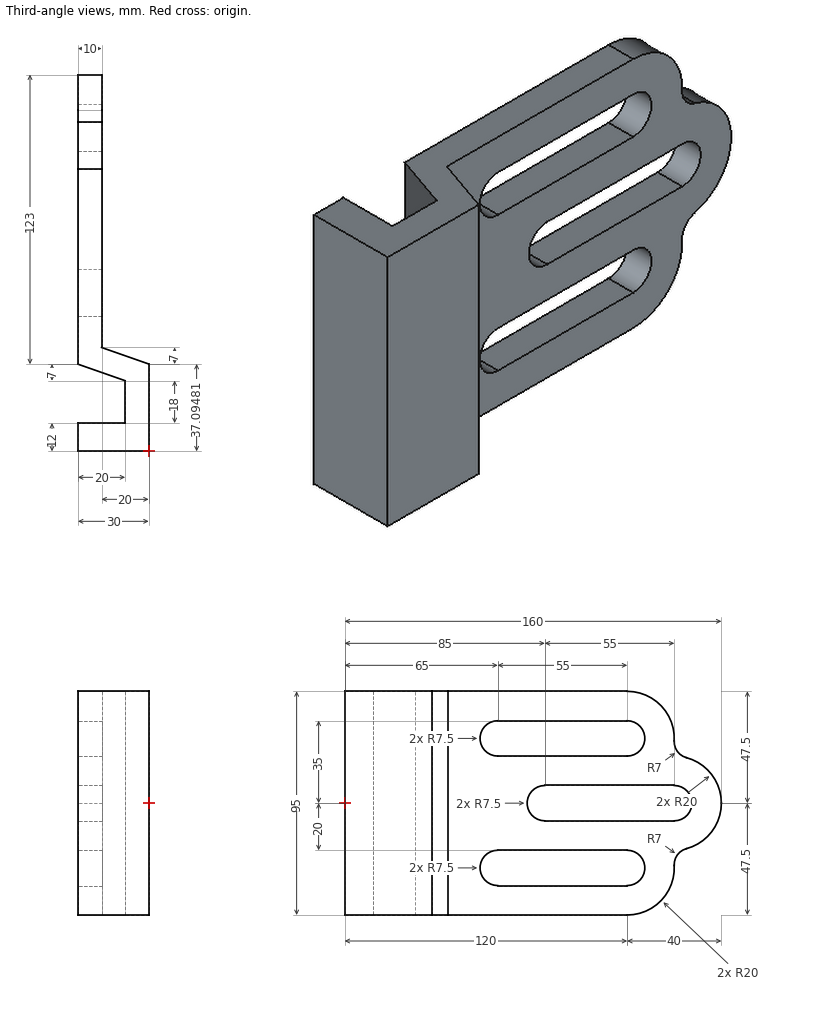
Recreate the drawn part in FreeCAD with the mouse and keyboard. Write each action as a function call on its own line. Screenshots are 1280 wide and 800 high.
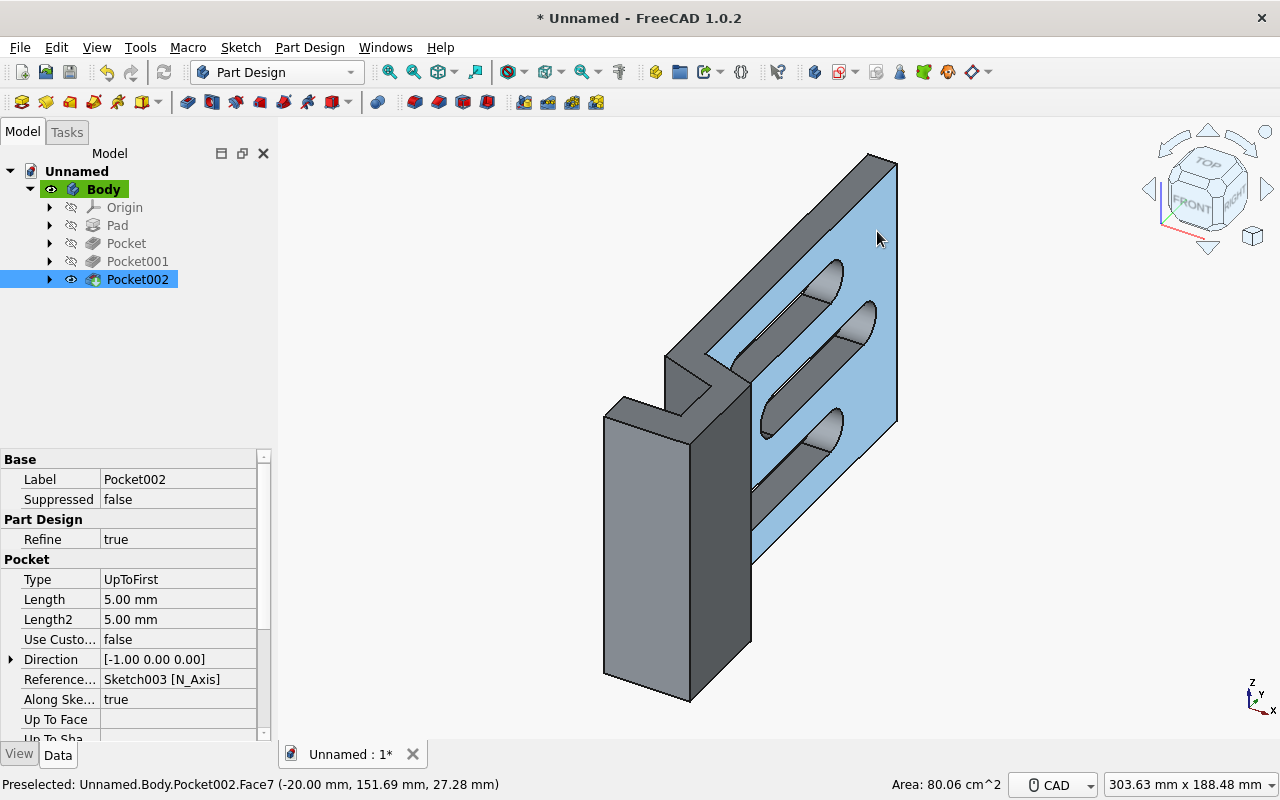
click(840, 72)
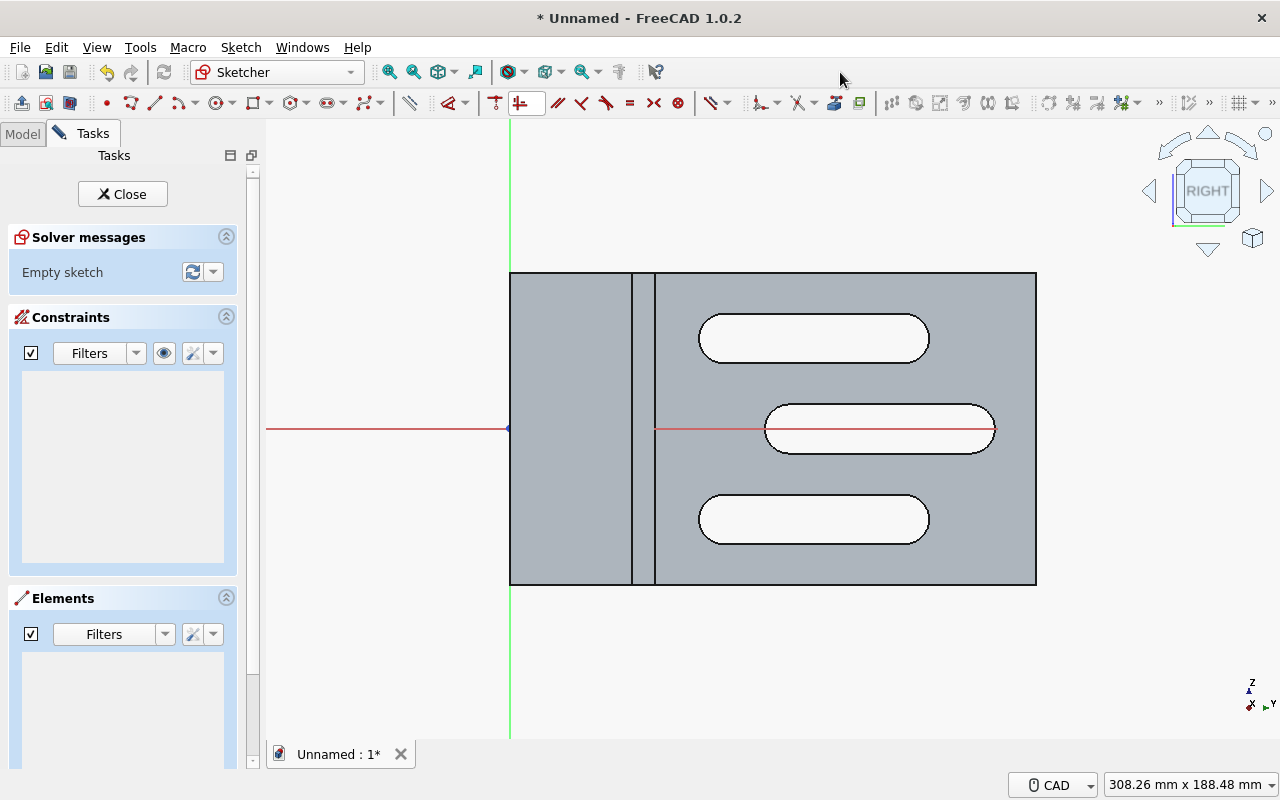
click(70, 104)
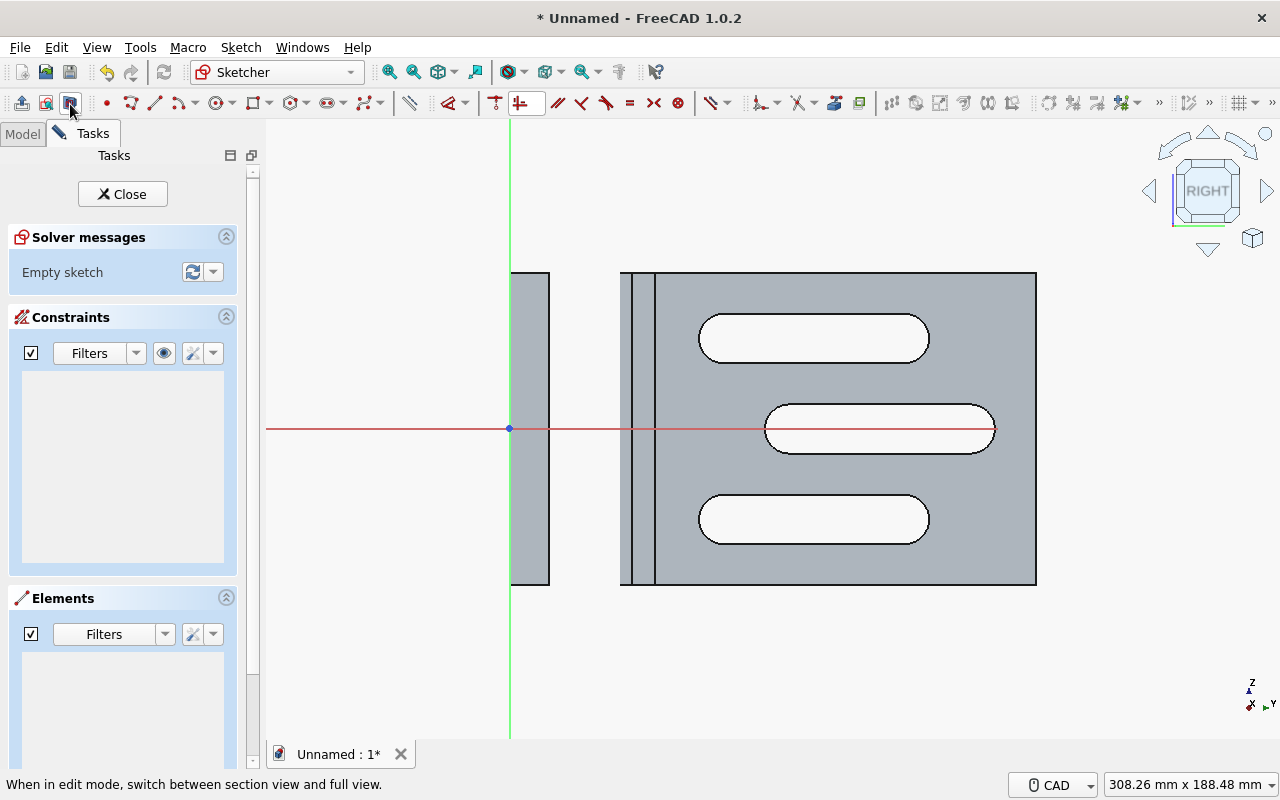
scroll(1115, 553, up, 5)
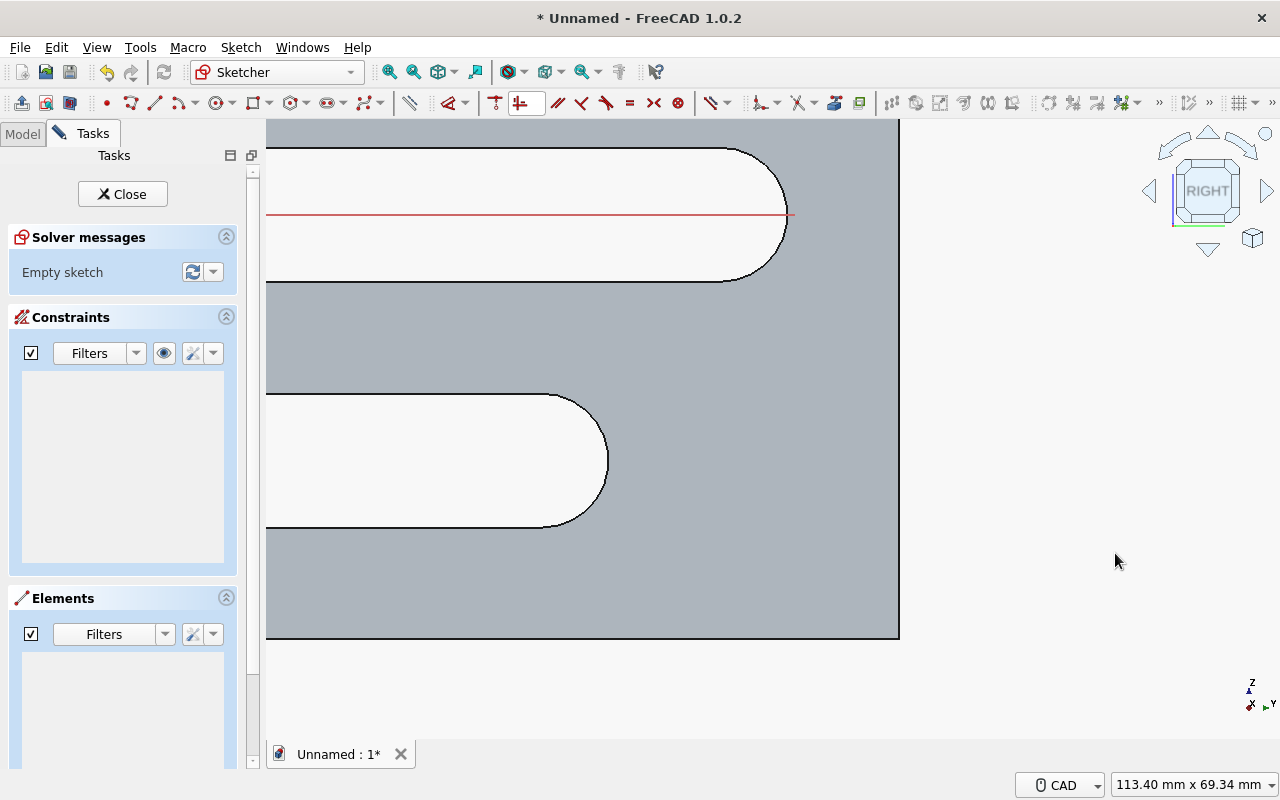
click(132, 104)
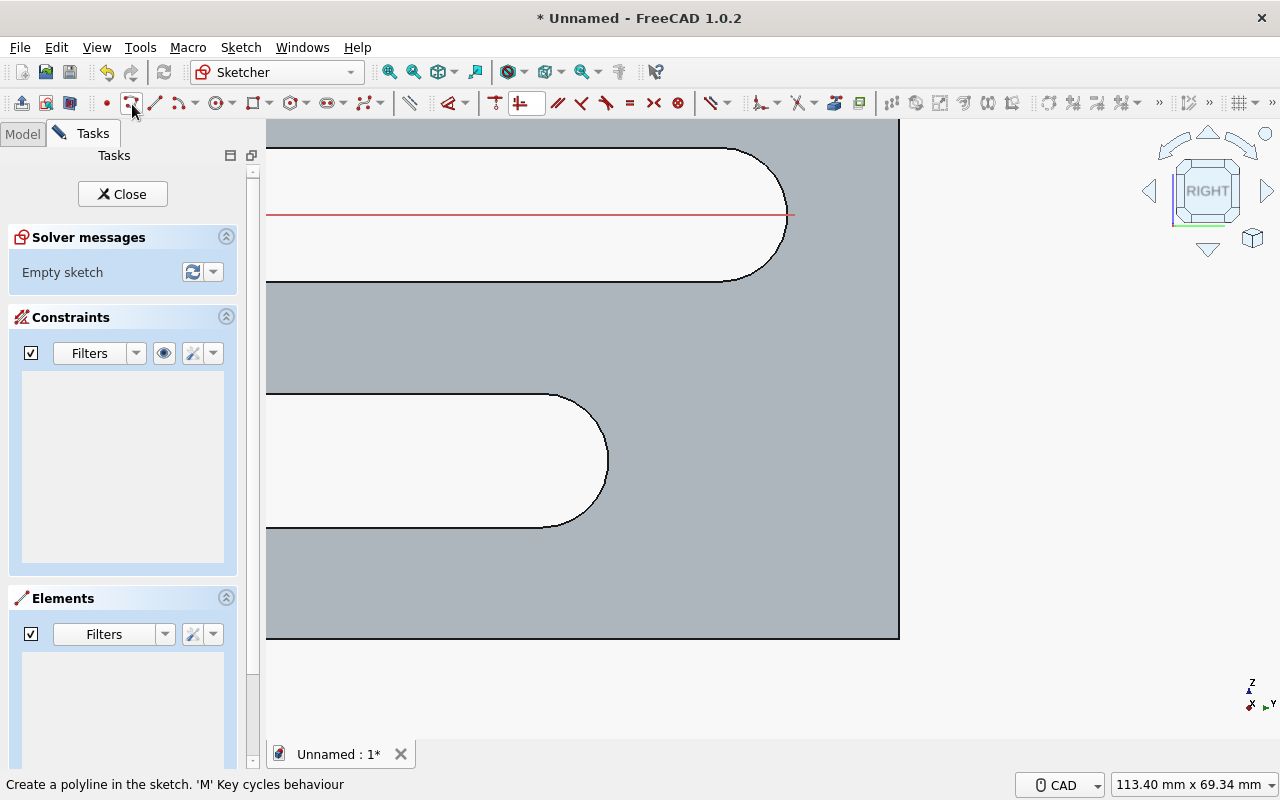
click(542, 639)
click(899, 639)
click(899, 215)
right_click(899, 215)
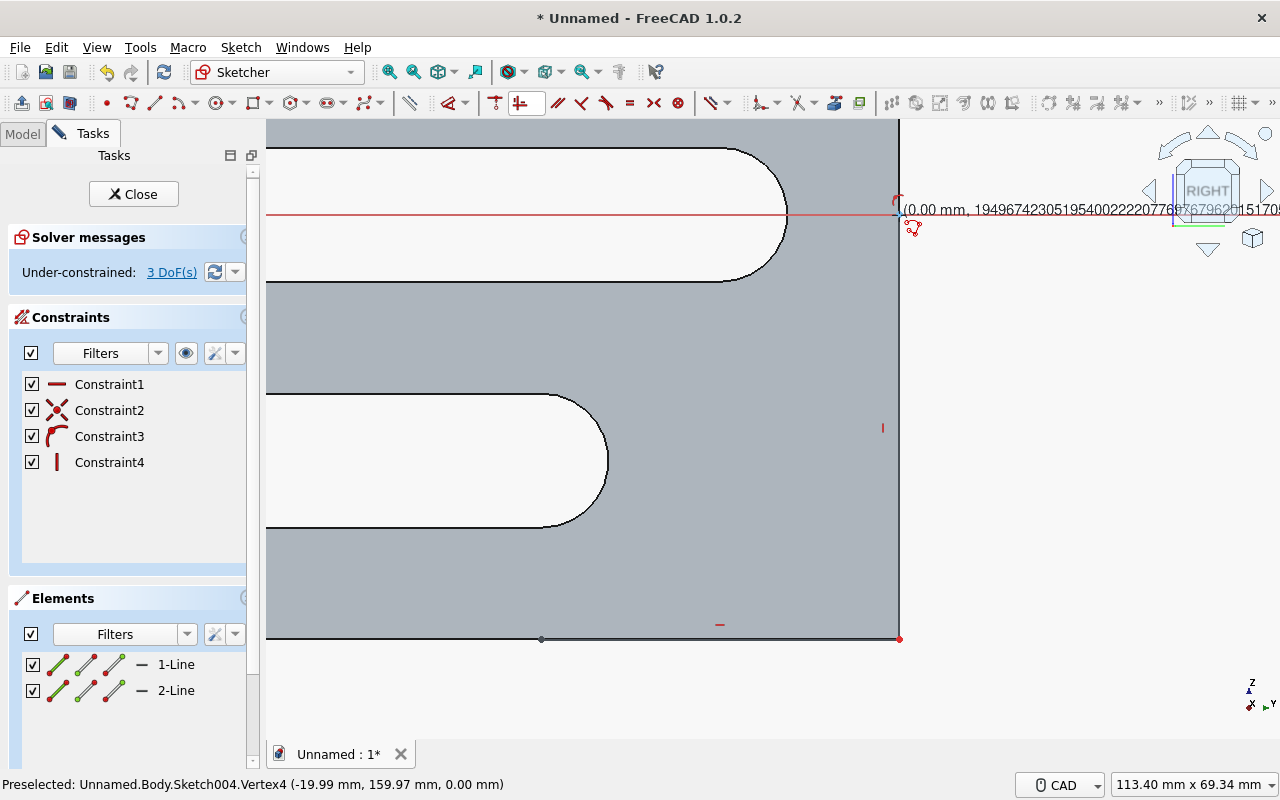
key(g)
key(3)
key(a)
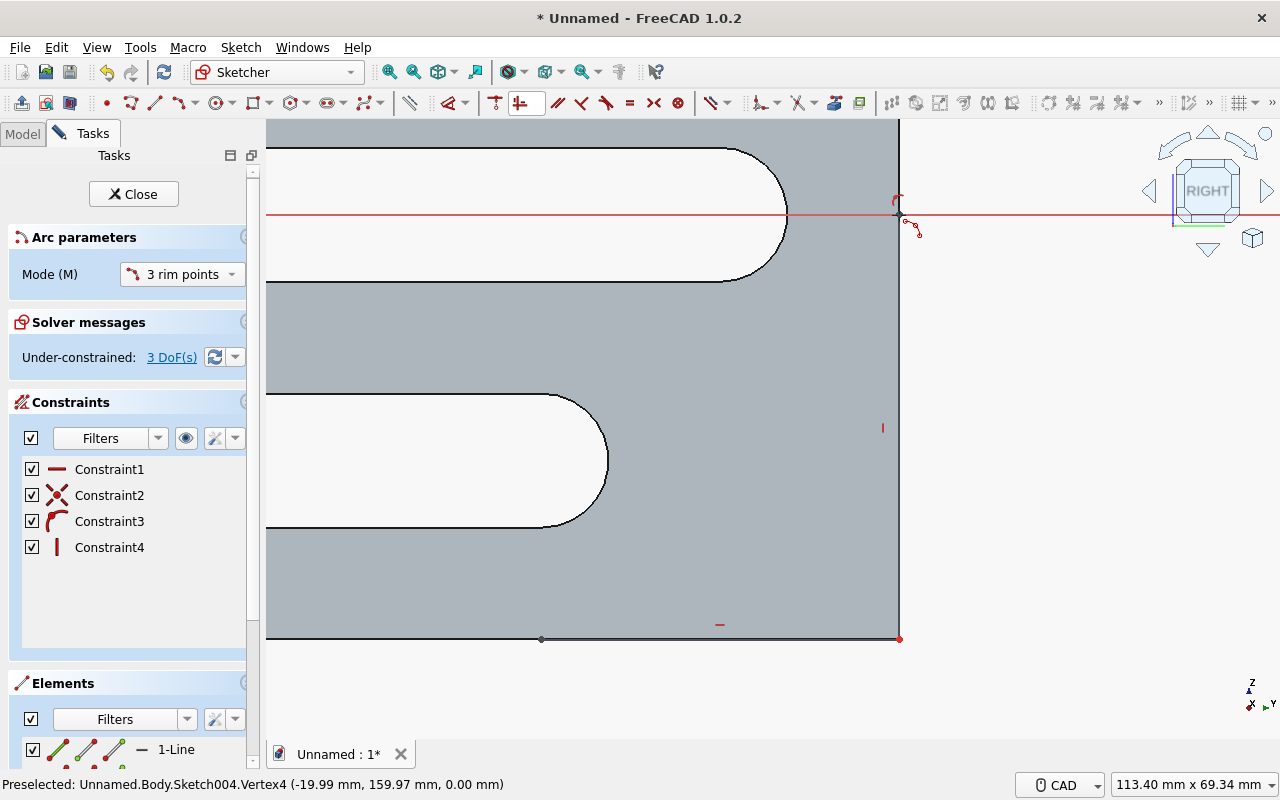
click(899, 215)
click(767, 388)
click(862, 324)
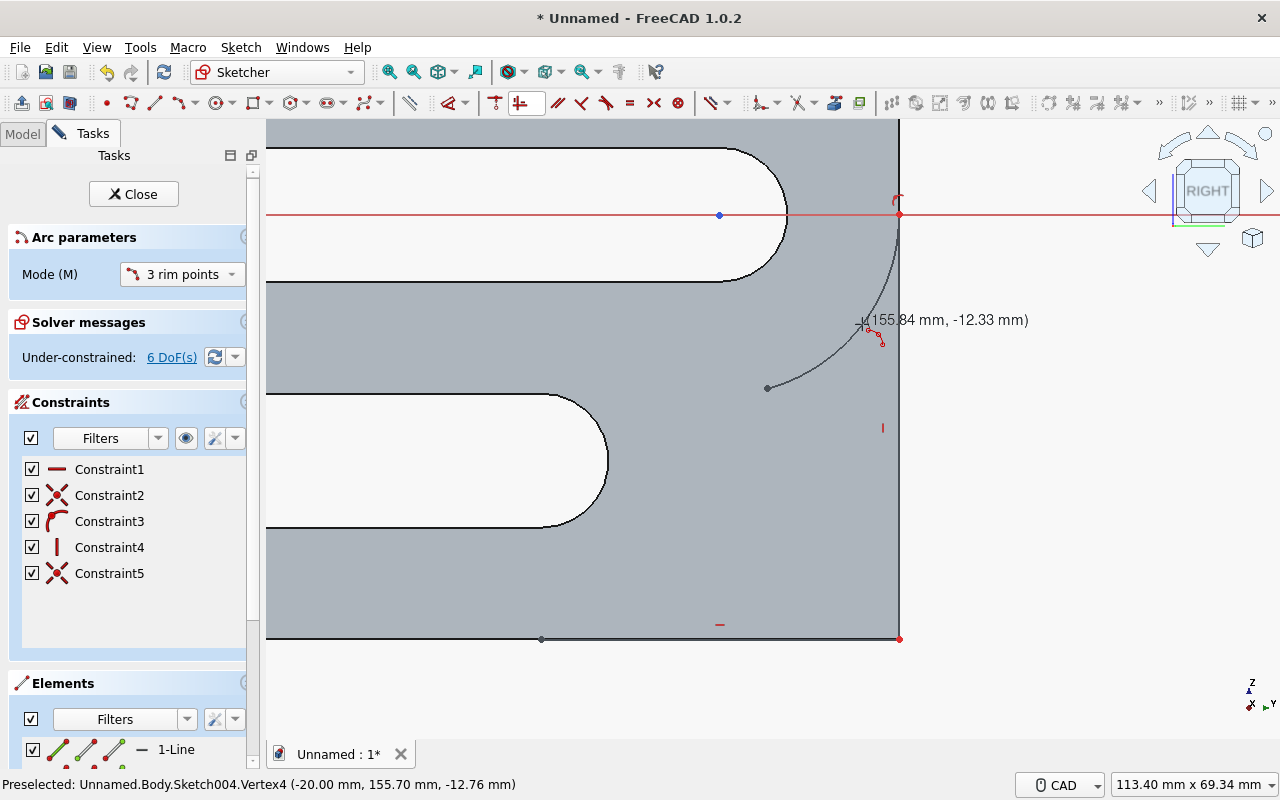
click(767, 389)
click(720, 451)
click(732, 411)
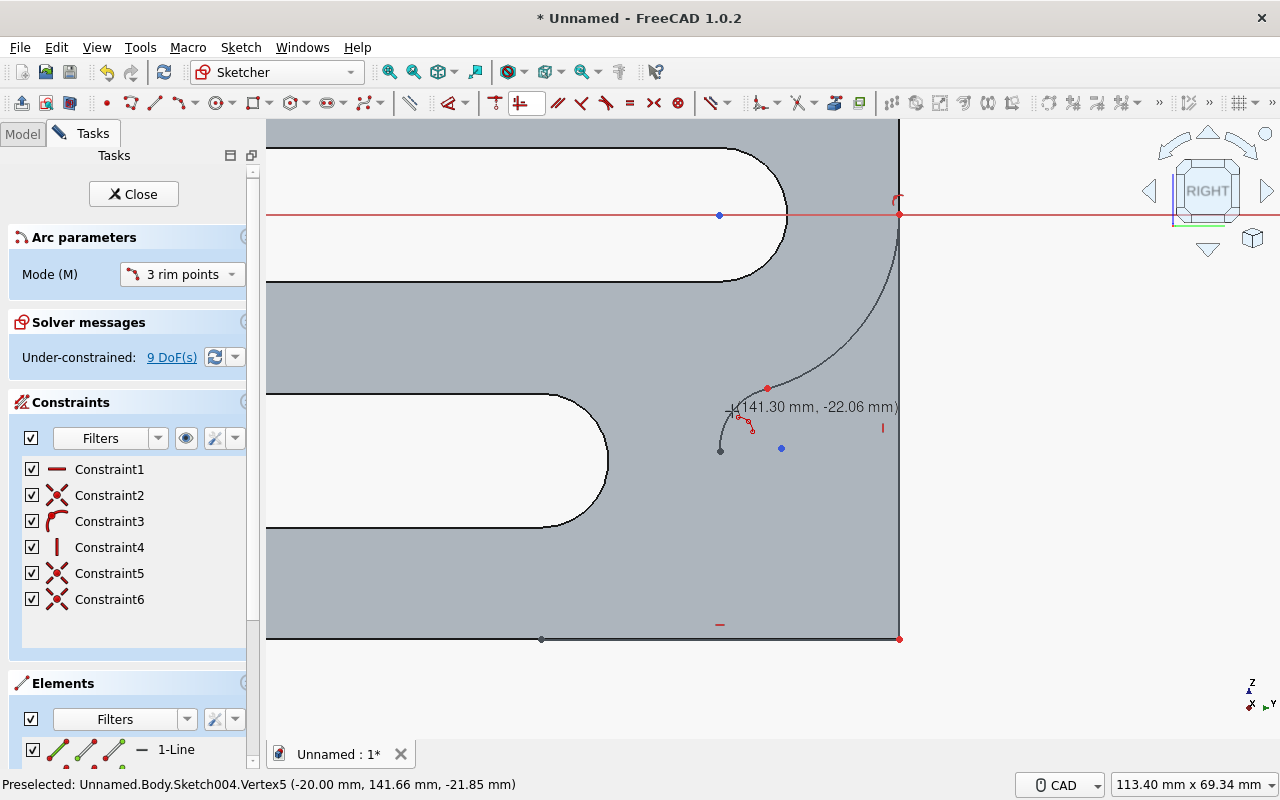
click(720, 452)
click(542, 640)
click(671, 584)
key(Escape)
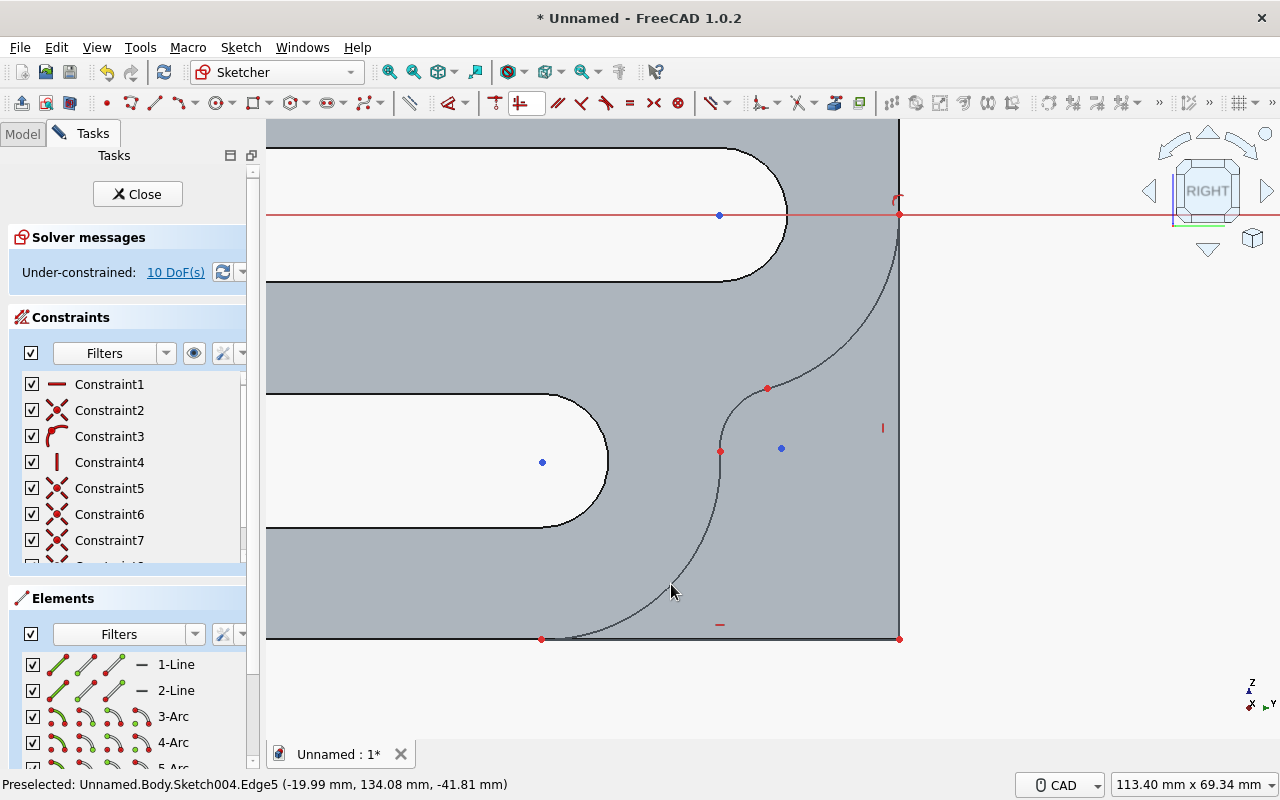
click(649, 640)